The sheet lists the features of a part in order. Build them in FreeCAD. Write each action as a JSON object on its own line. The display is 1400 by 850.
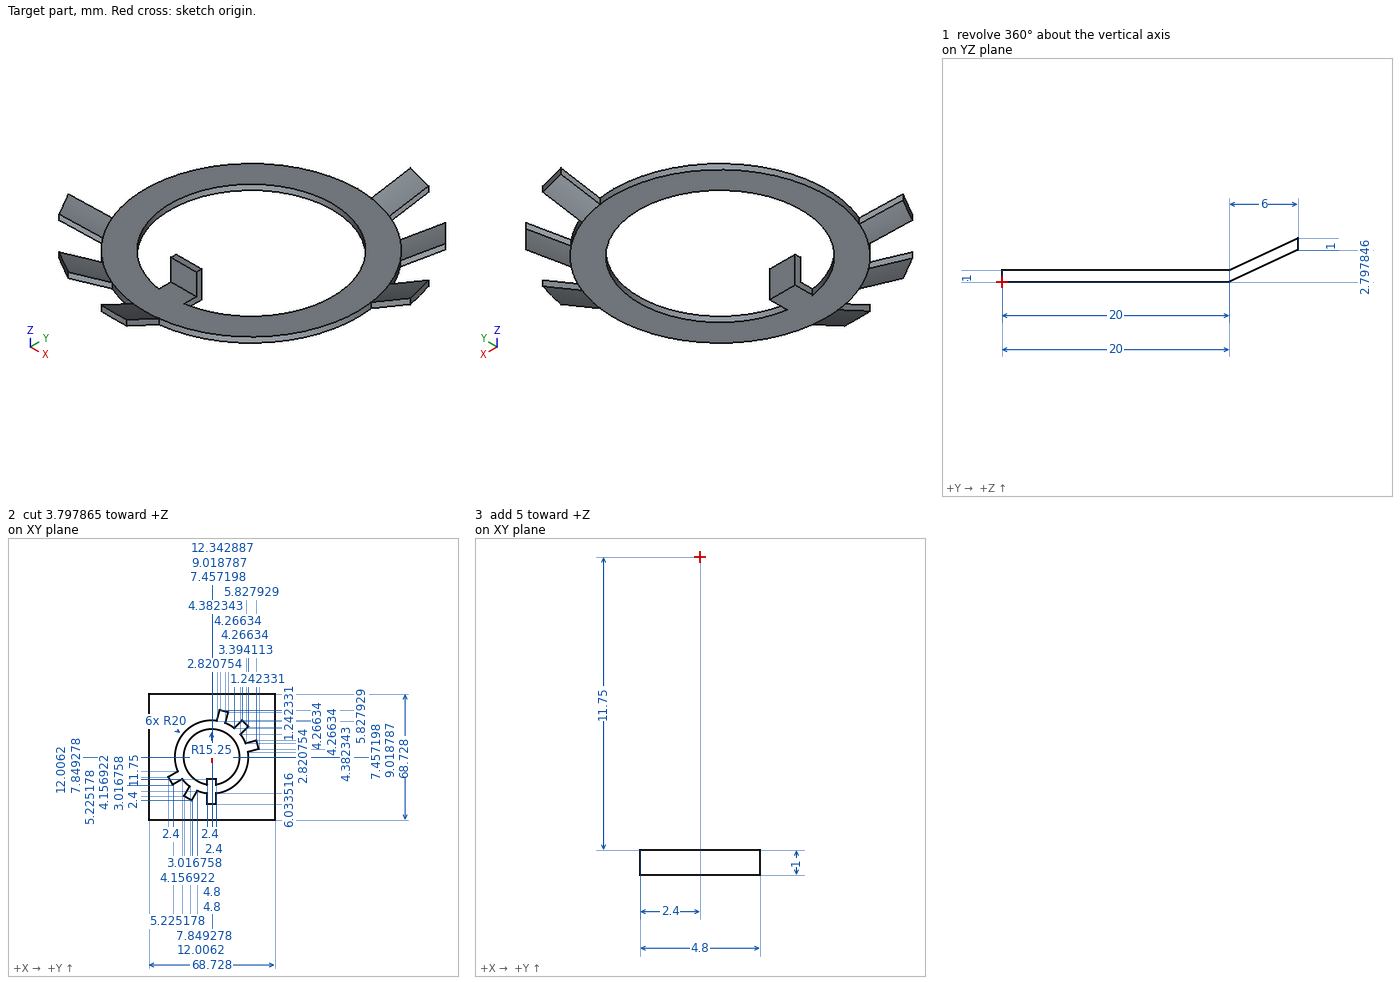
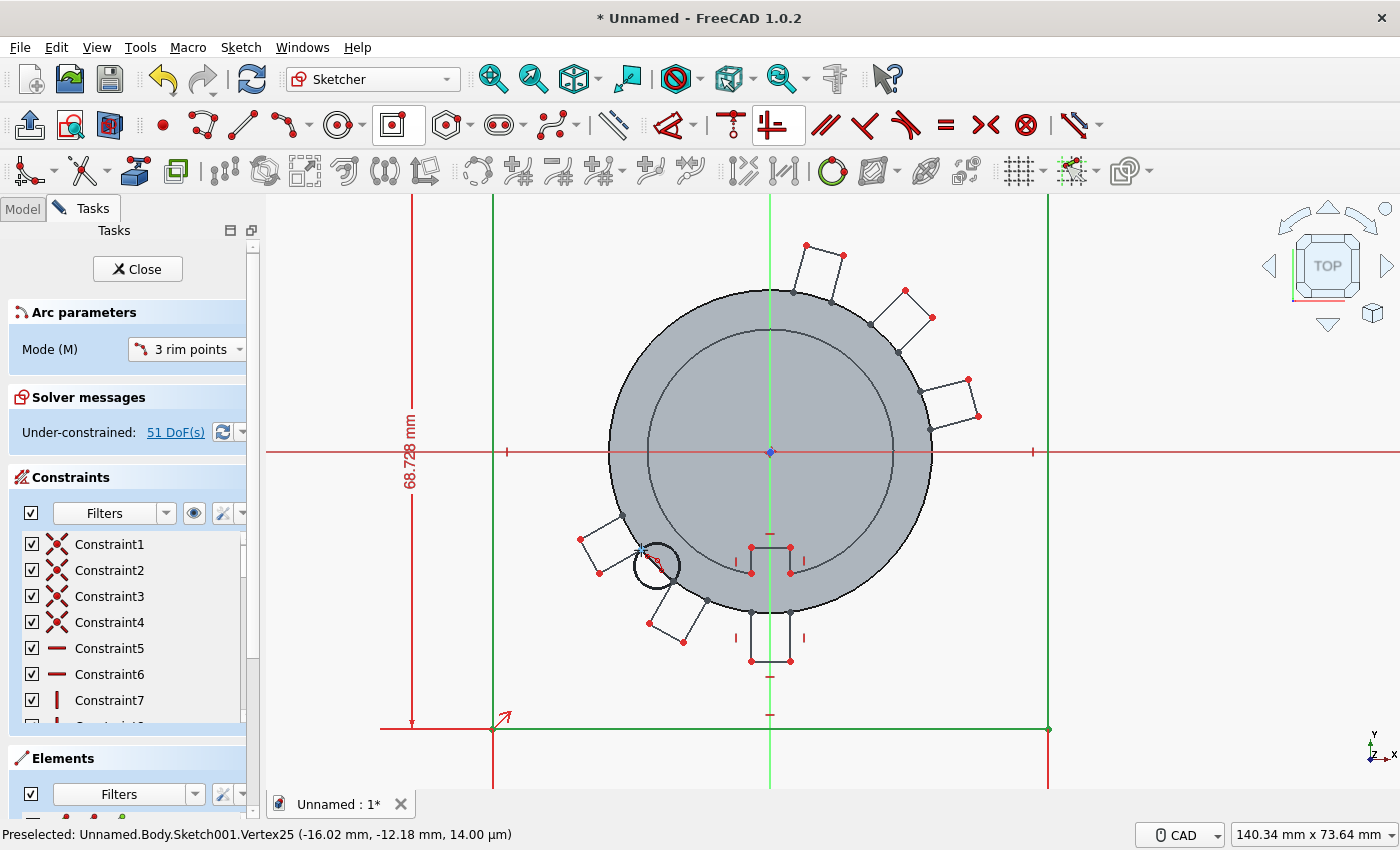
{"action": "scroll", "coordinate": [656, 566], "scroll_direction": "up", "scroll_amount": 12}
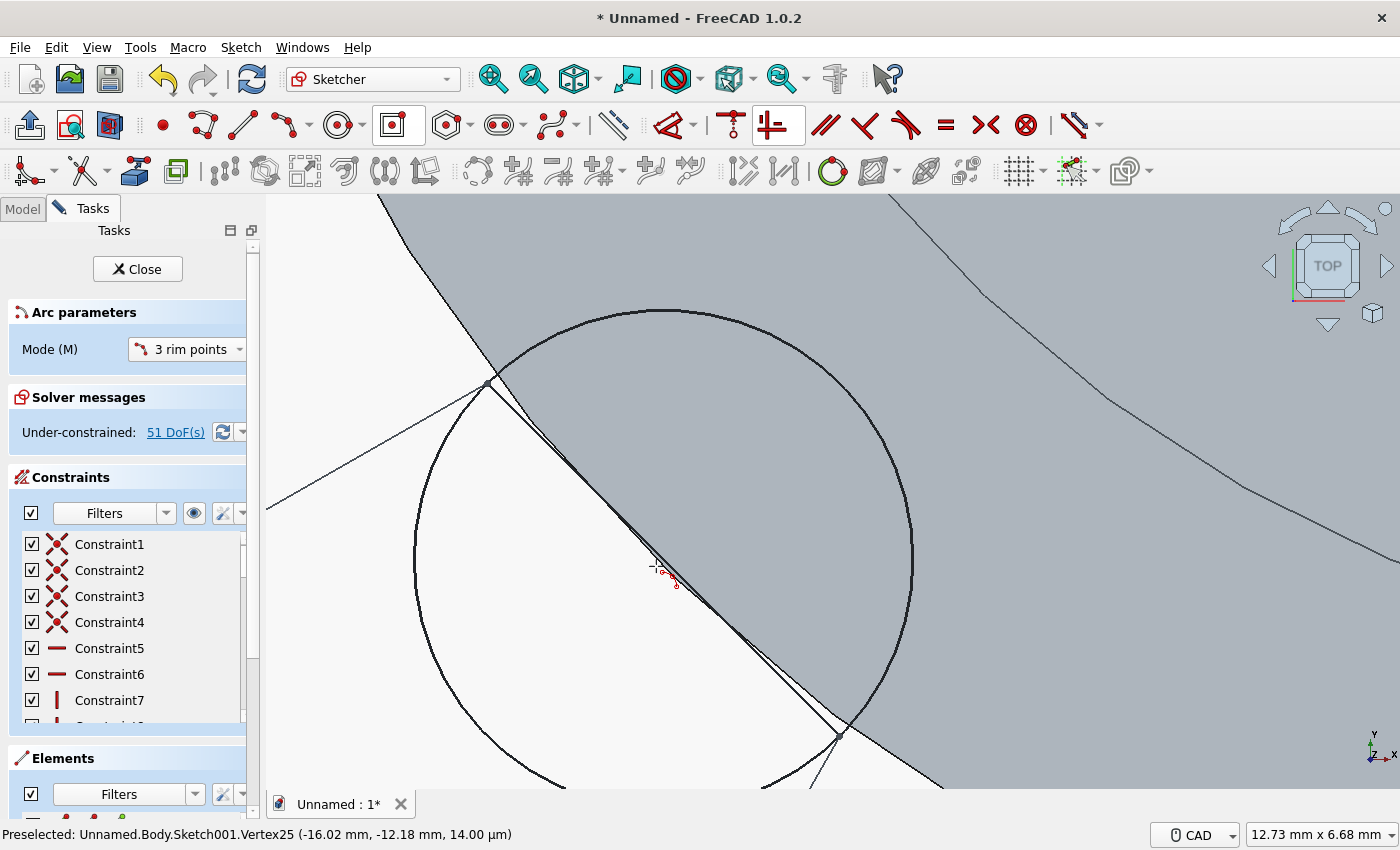
{"action": "left_click", "coordinate": [655, 558]}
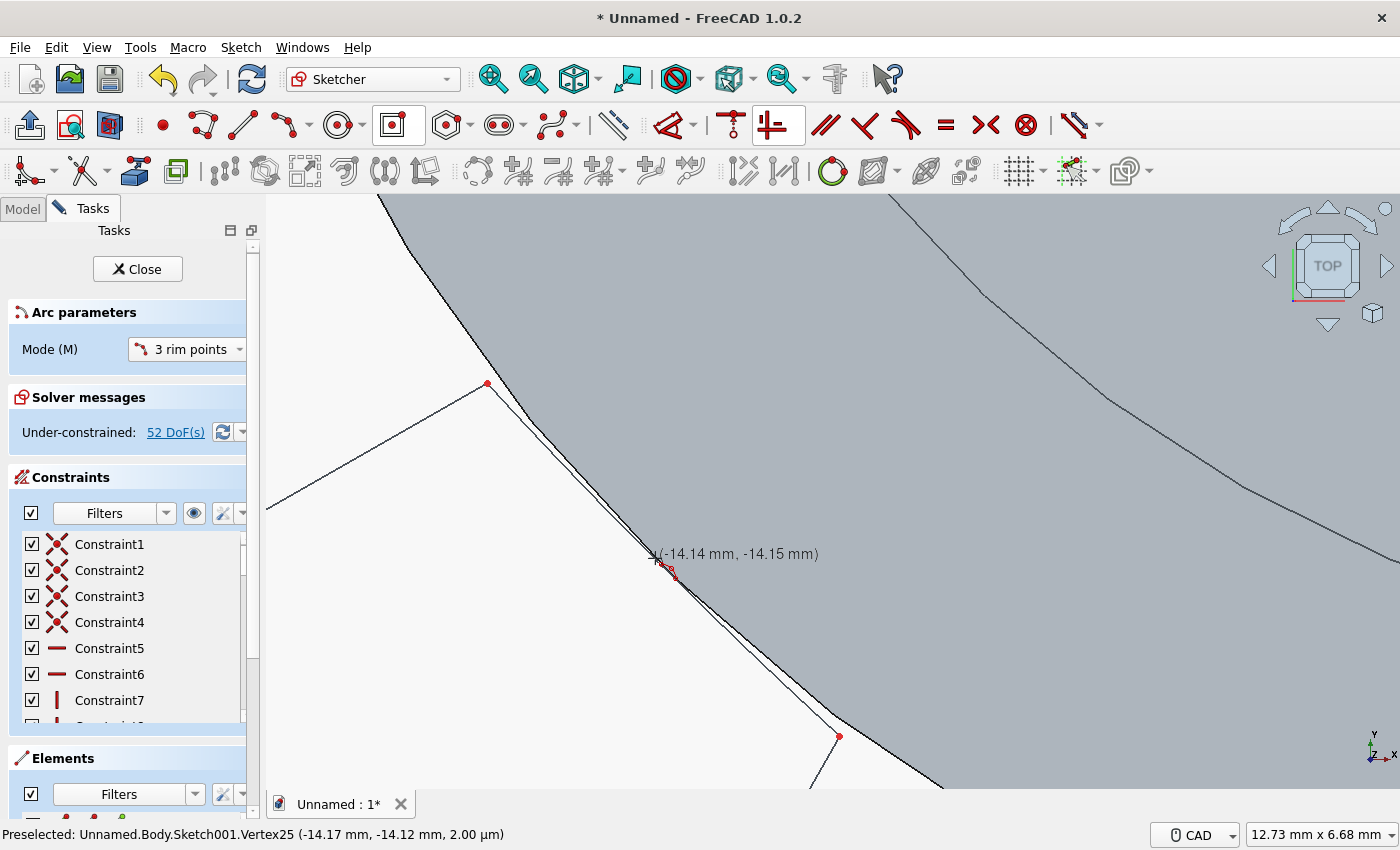
{"action": "scroll", "coordinate": [690, 569], "scroll_direction": "down", "scroll_amount": 14}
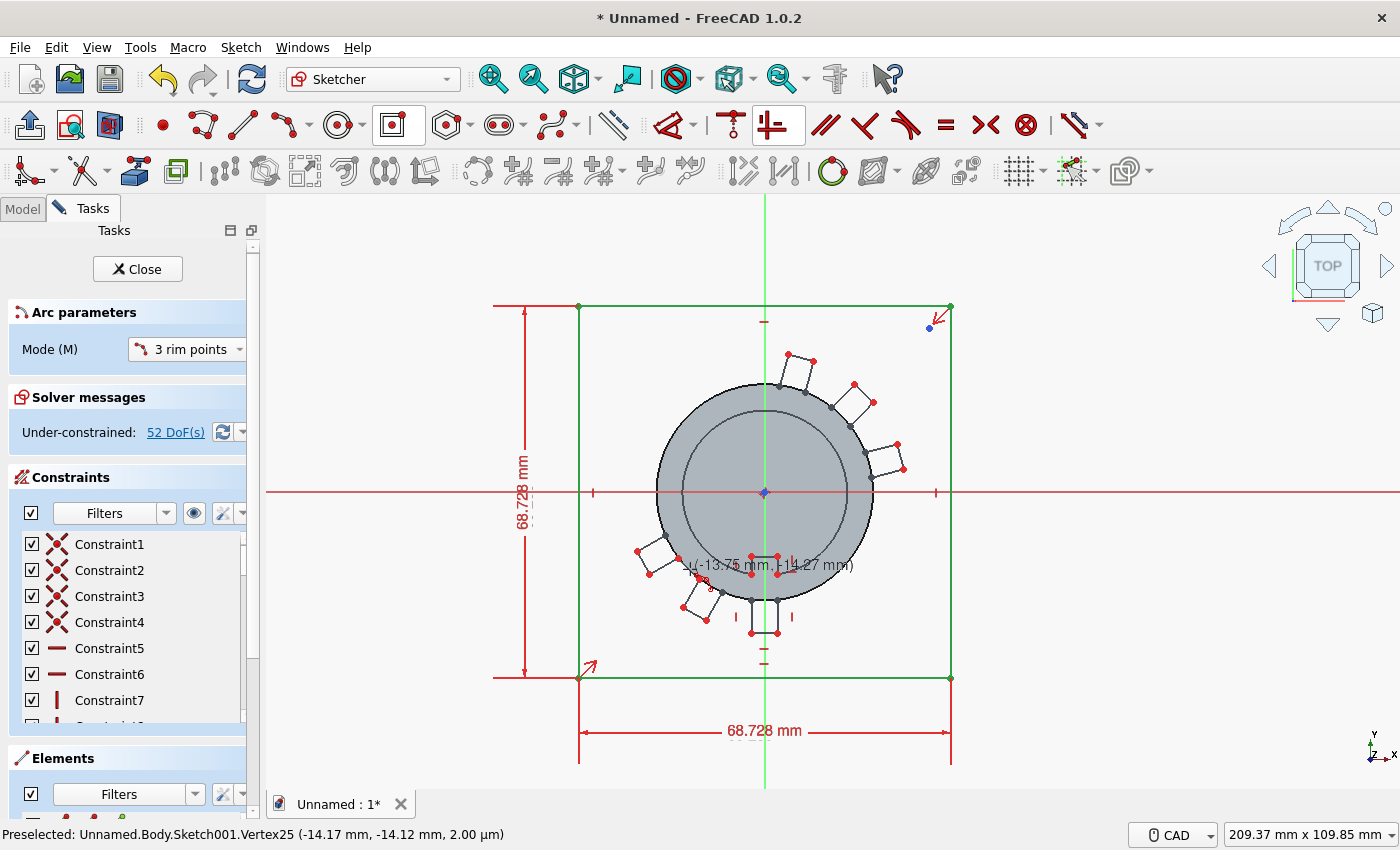
{"action": "left_click", "coordinate": [665, 536]}
{"action": "left_click", "coordinate": [780, 386]}
{"action": "left_click", "coordinate": [679, 426]}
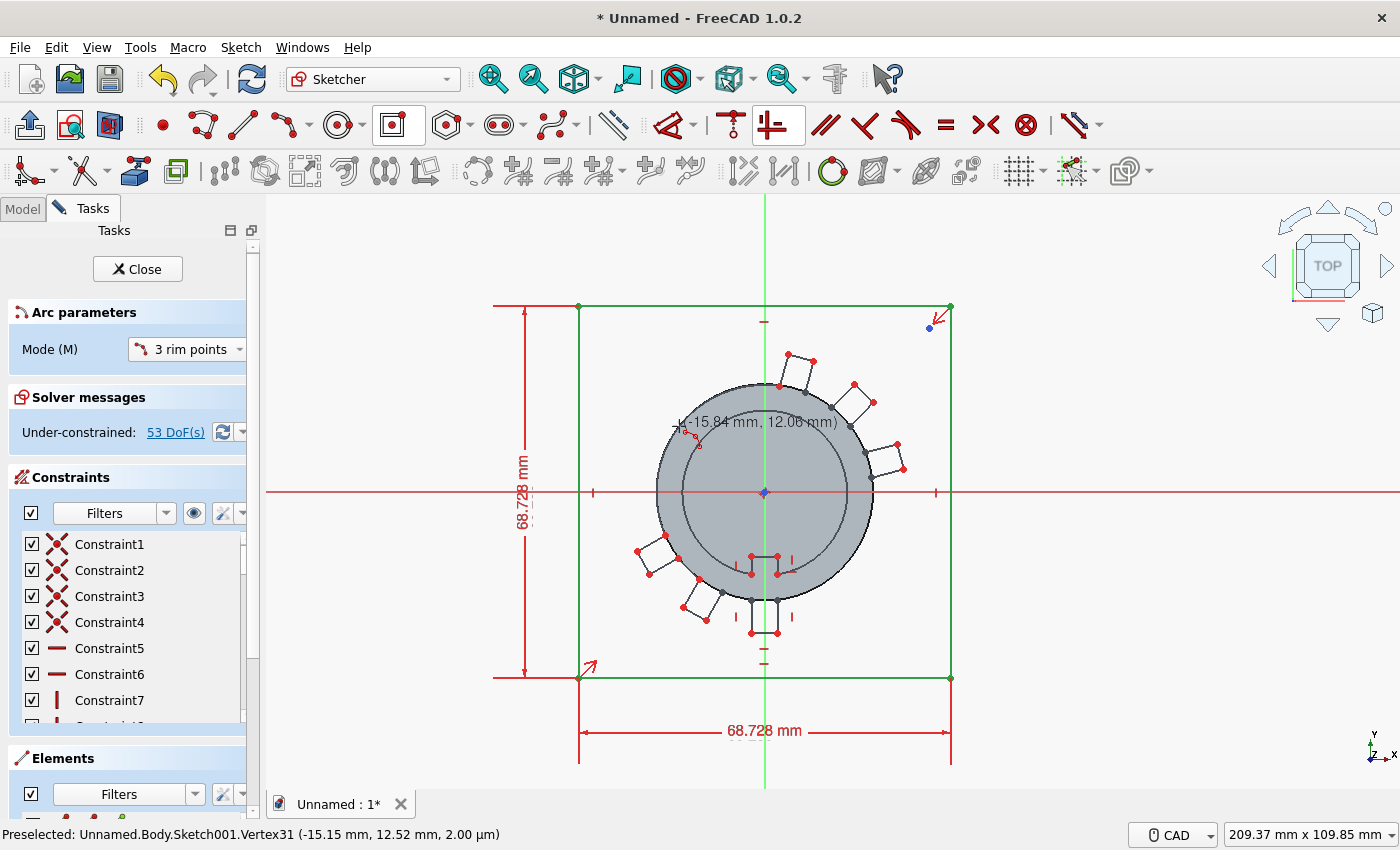
{"action": "left_click", "coordinate": [805, 393]}
{"action": "left_click", "coordinate": [832, 407]}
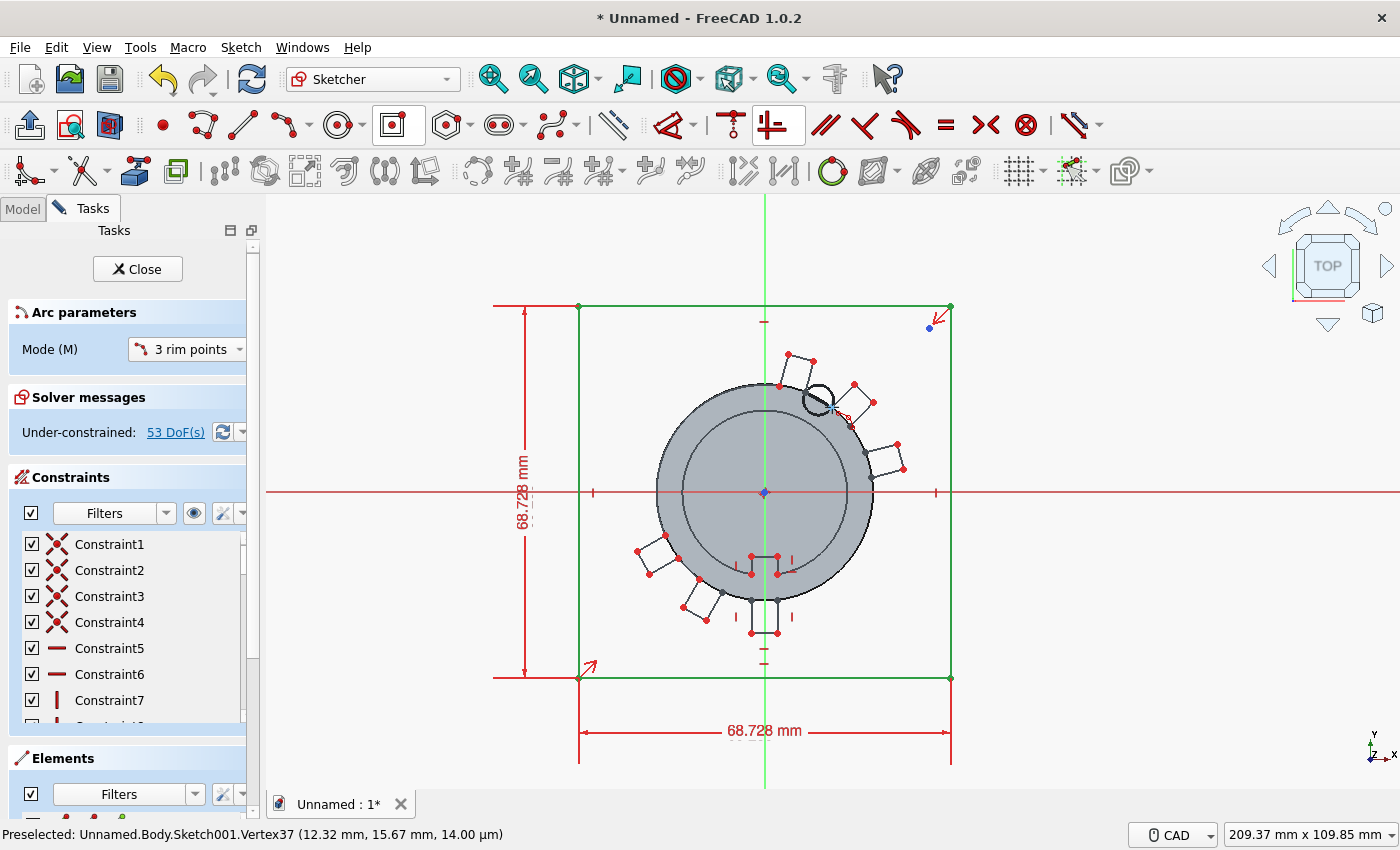
{"action": "scroll", "coordinate": [819, 399], "scroll_direction": "up", "scroll_amount": 14}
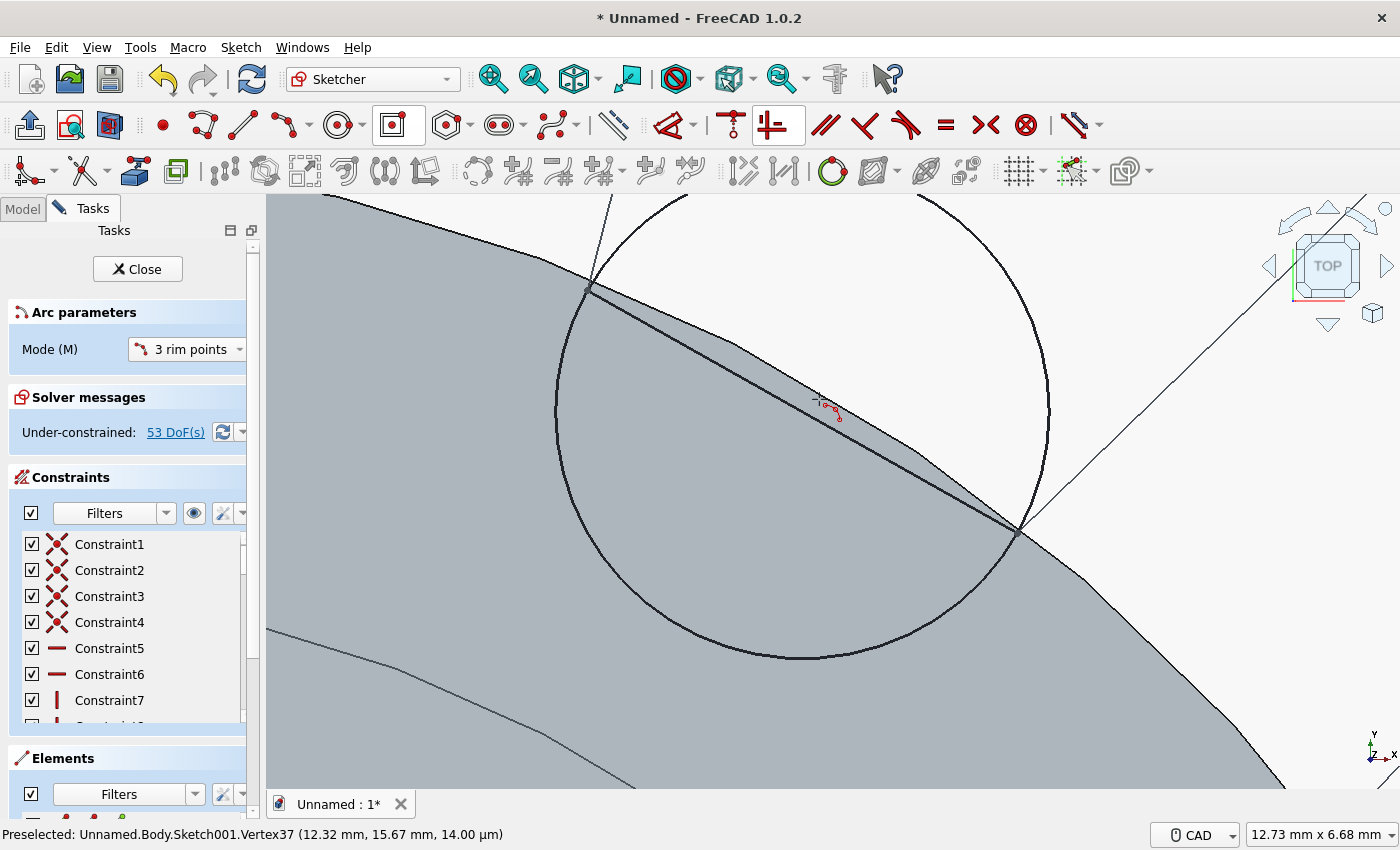
{"action": "left_click", "coordinate": [811, 386]}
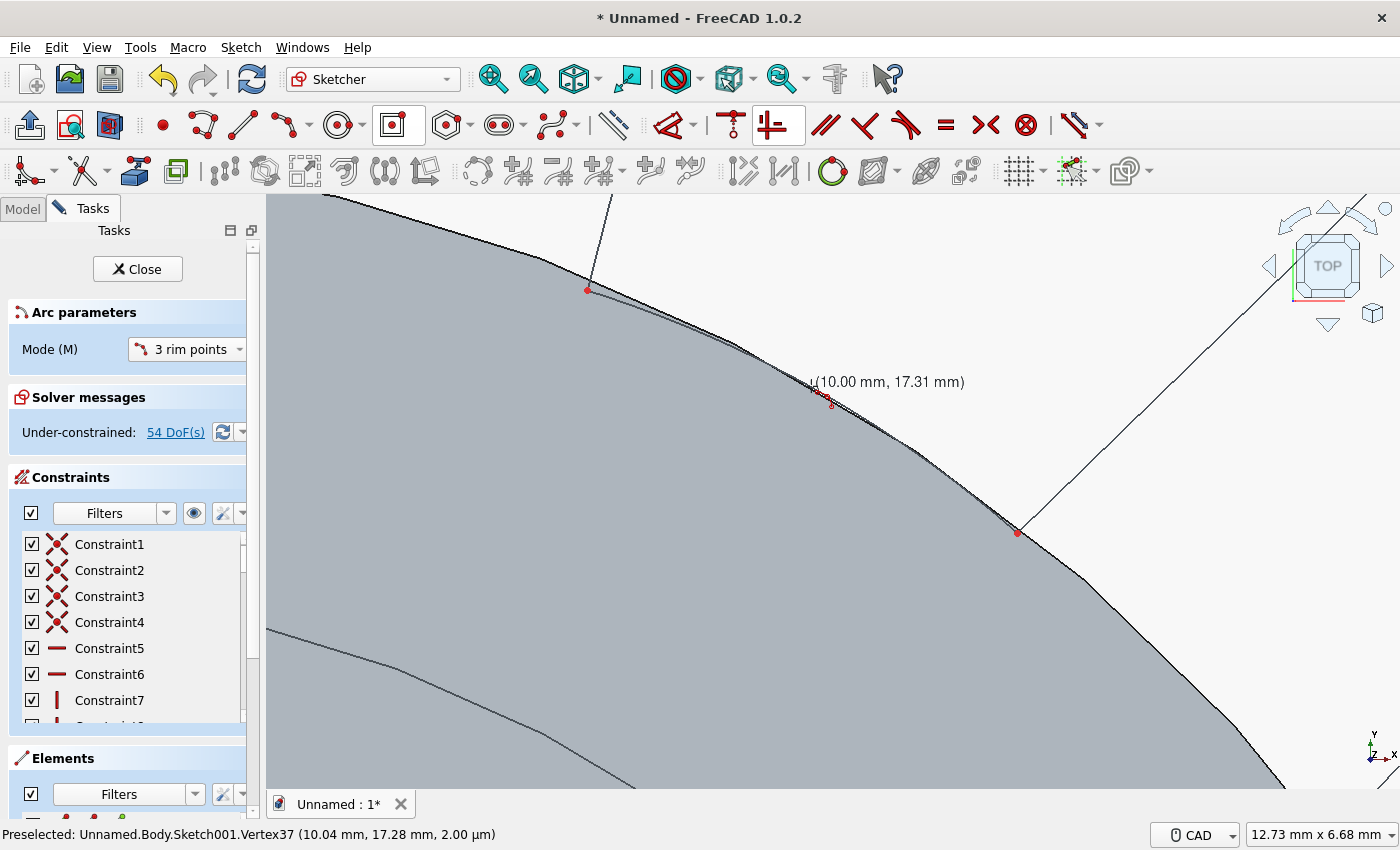
{"action": "scroll", "coordinate": [819, 398], "scroll_direction": "down", "scroll_amount": 14}